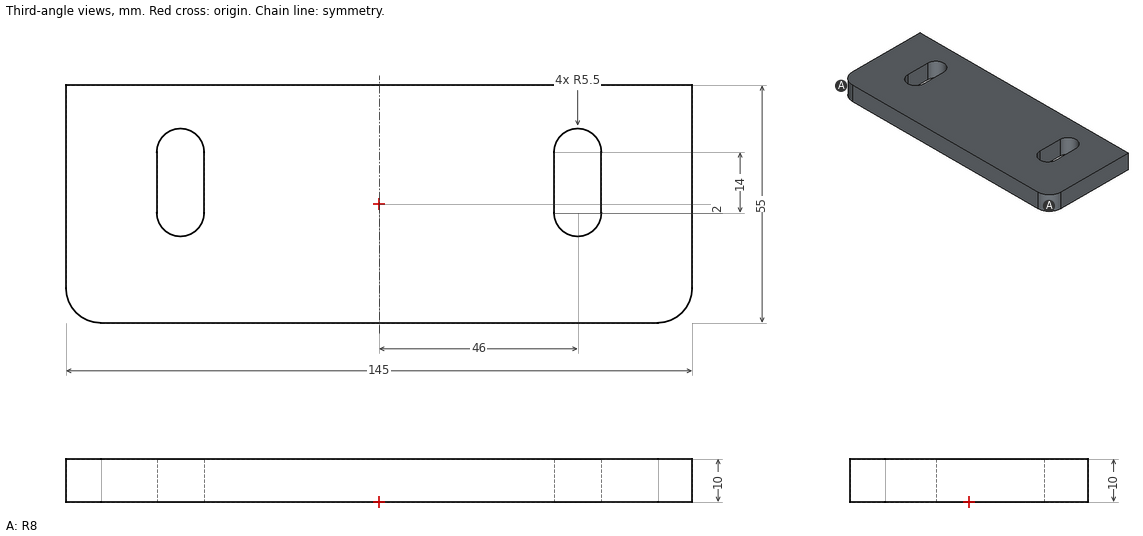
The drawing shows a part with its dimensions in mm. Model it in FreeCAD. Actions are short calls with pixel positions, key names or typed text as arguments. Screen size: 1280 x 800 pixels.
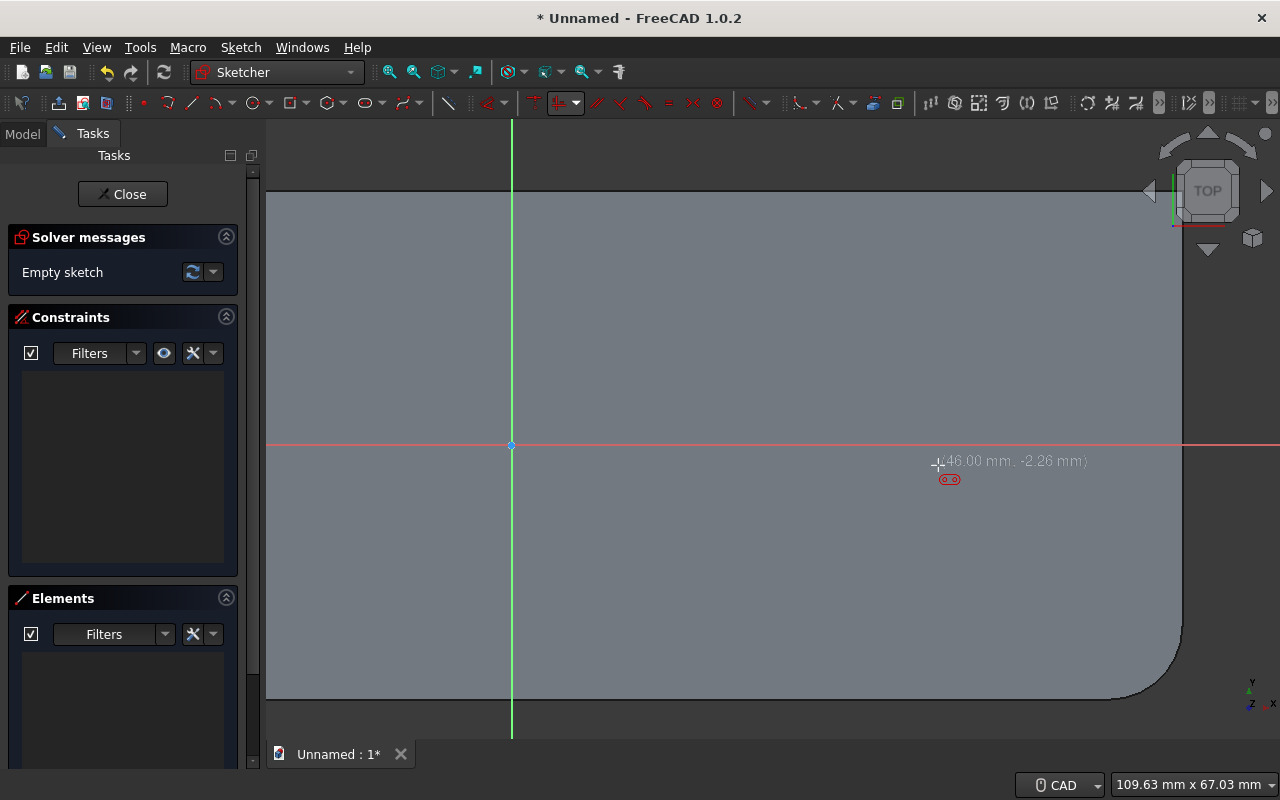
click(937, 464)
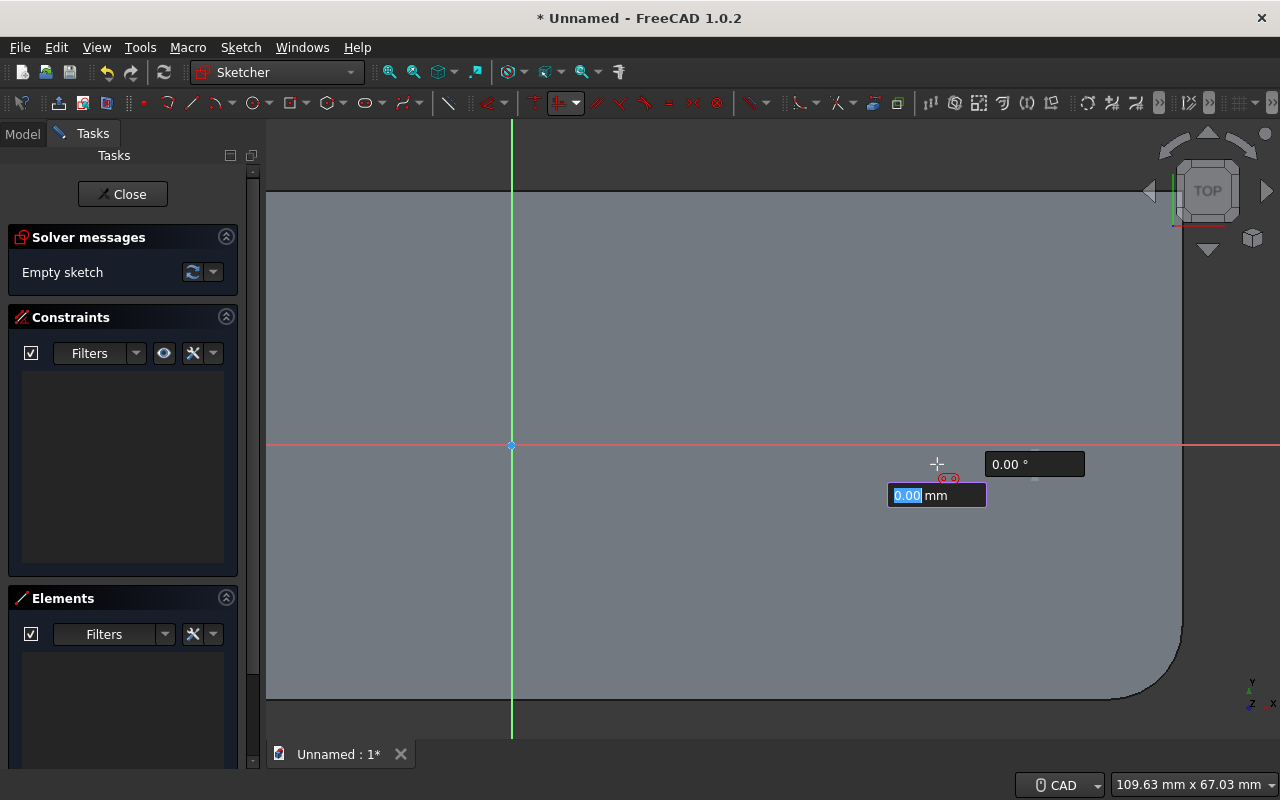
click(937, 334)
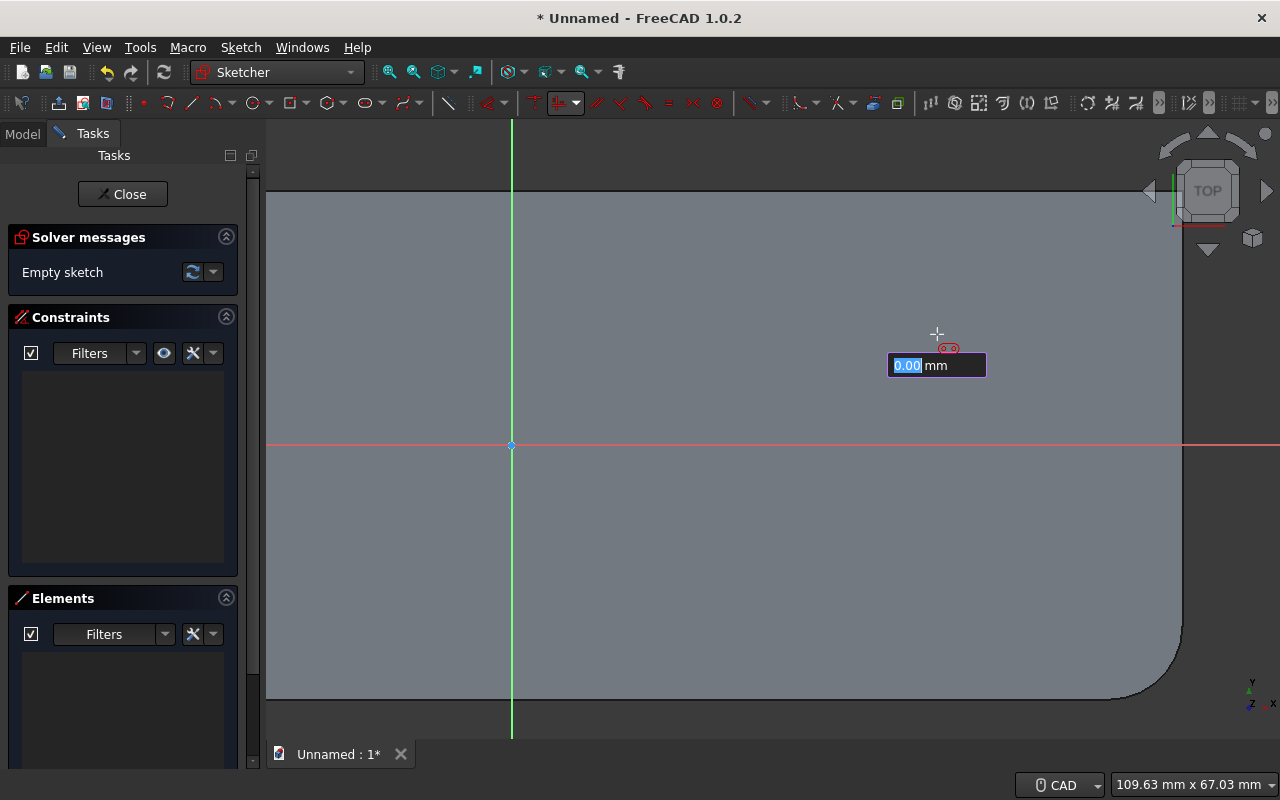
click(988, 399)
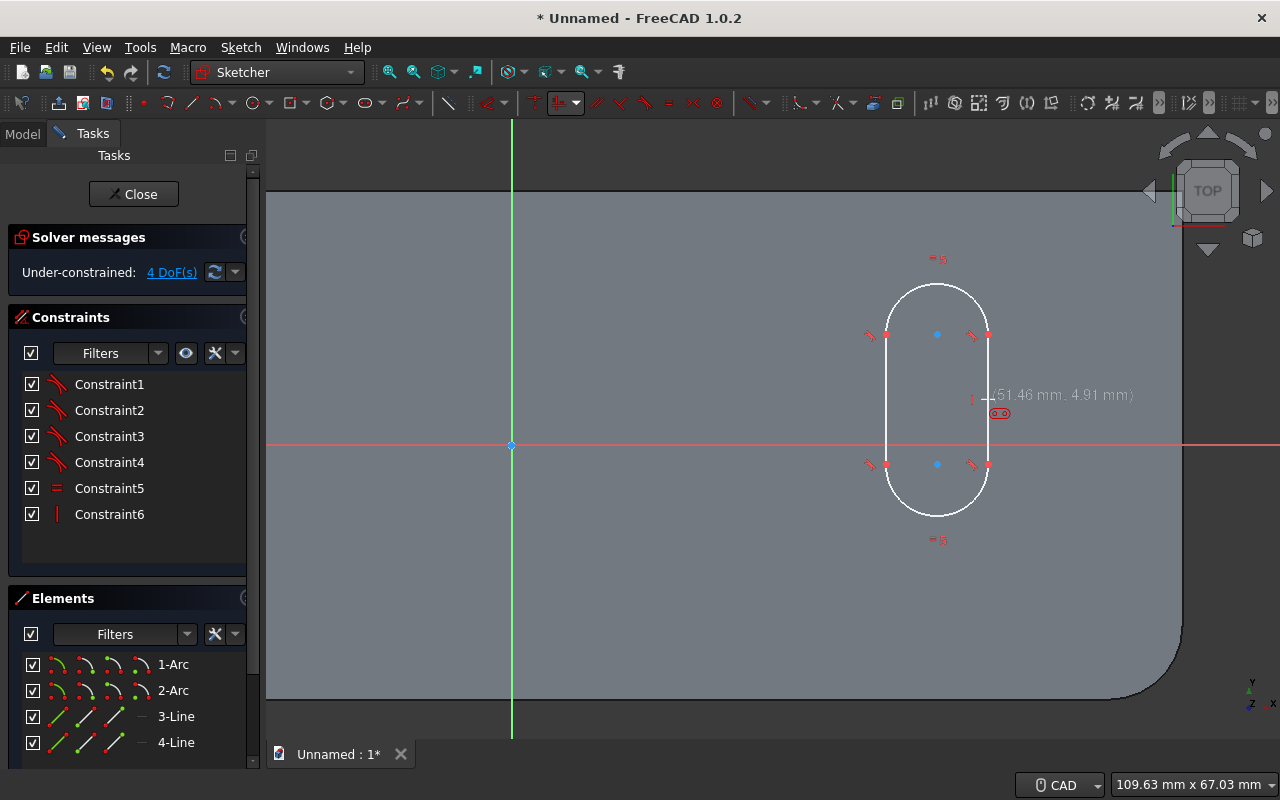
scroll(1096, 490, down, 2)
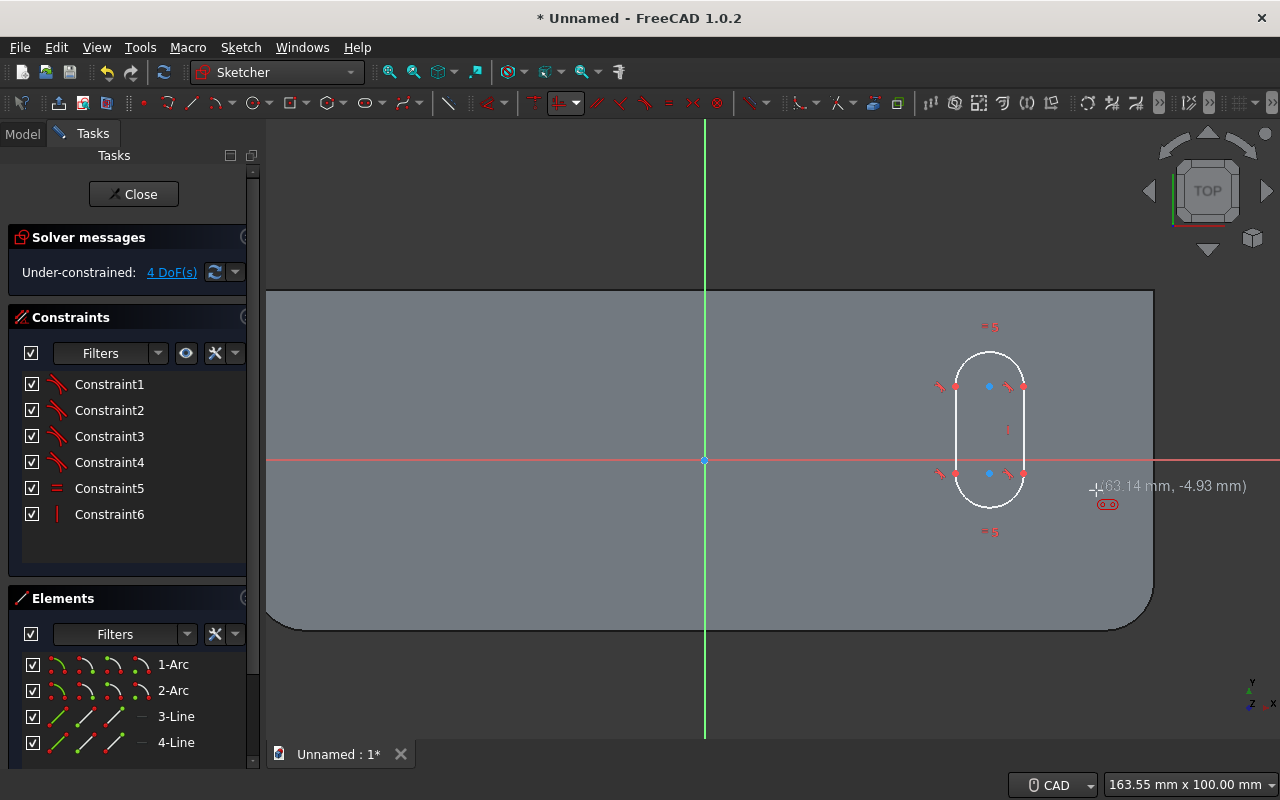
scroll(420, 473, up, 2)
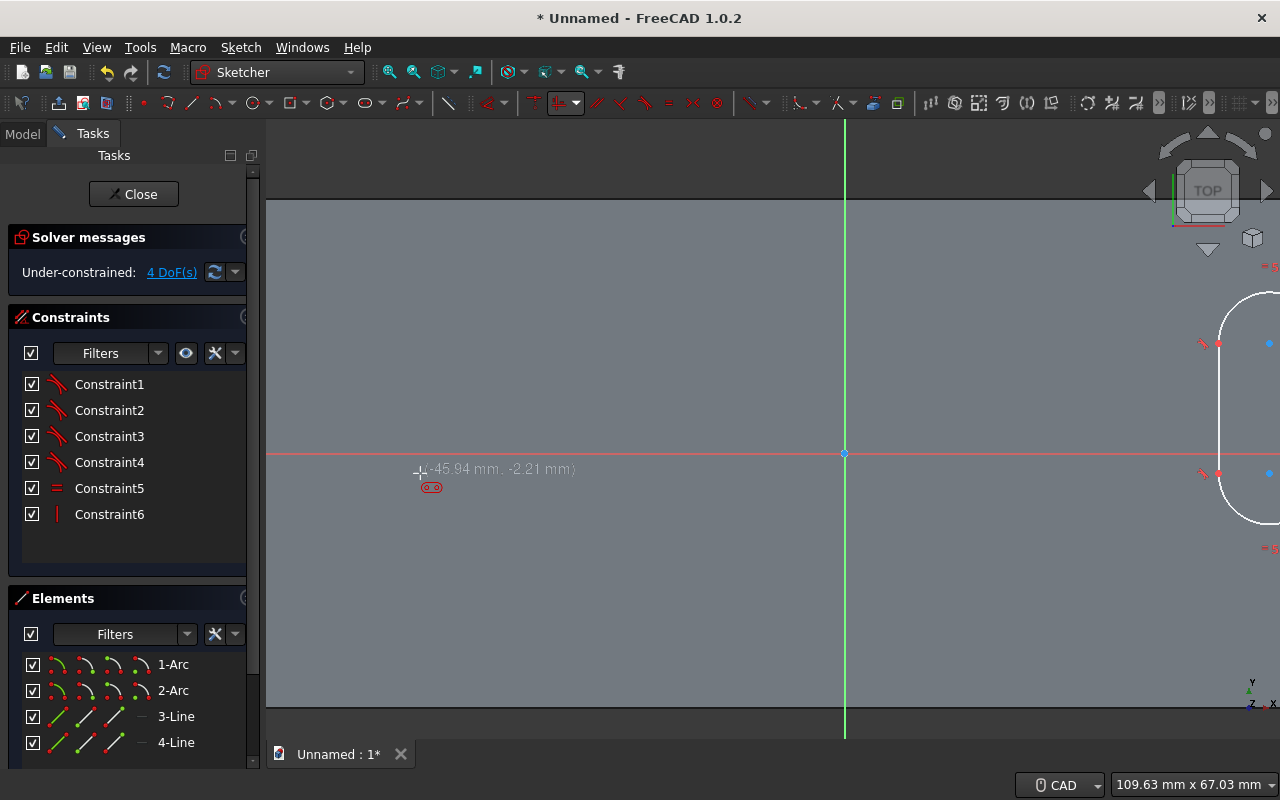
click(419, 472)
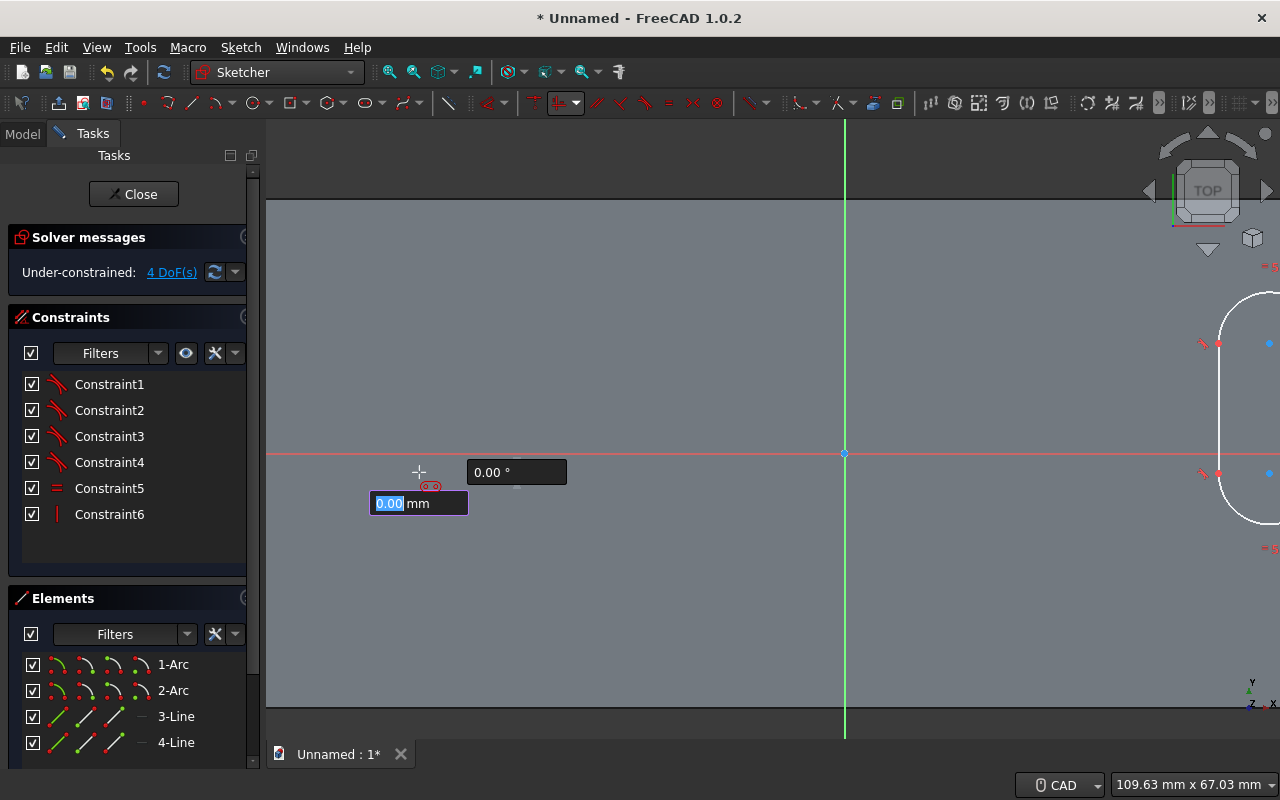
click(419, 343)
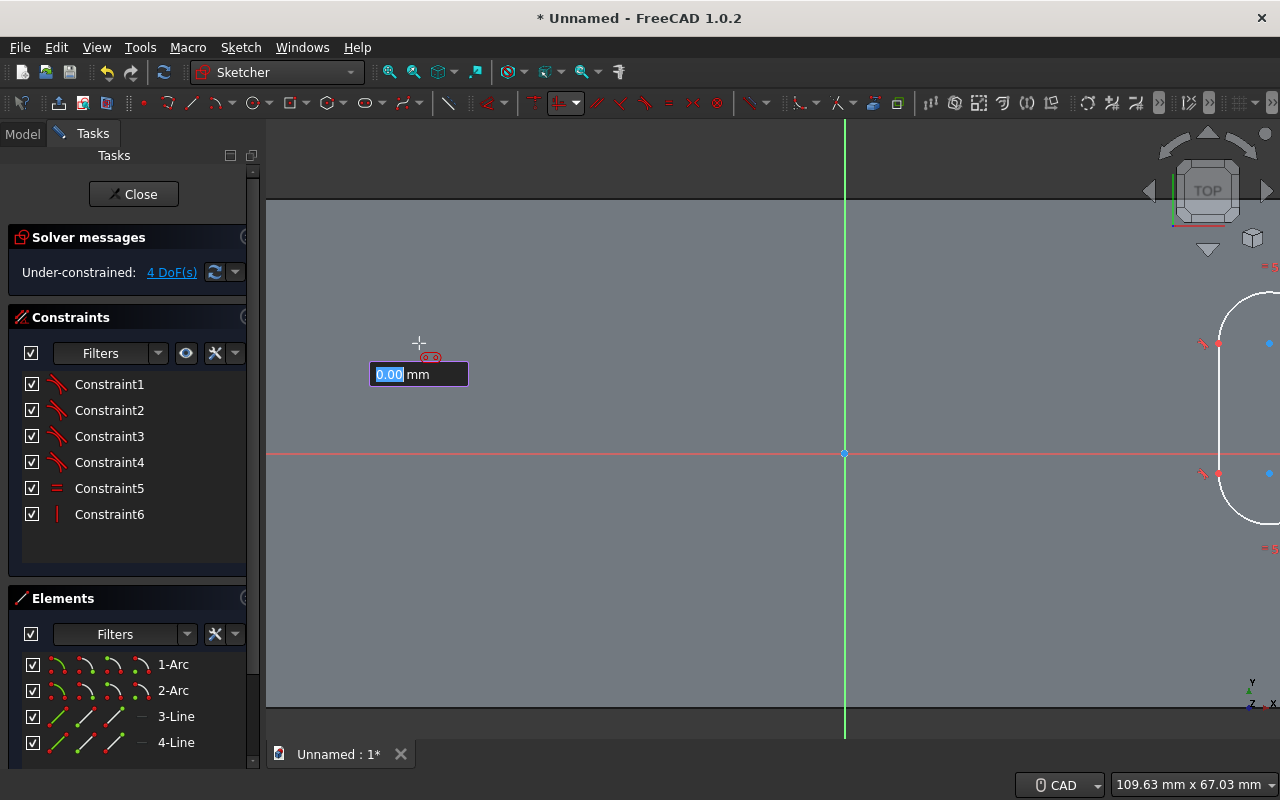
click(470, 408)
key(Escape)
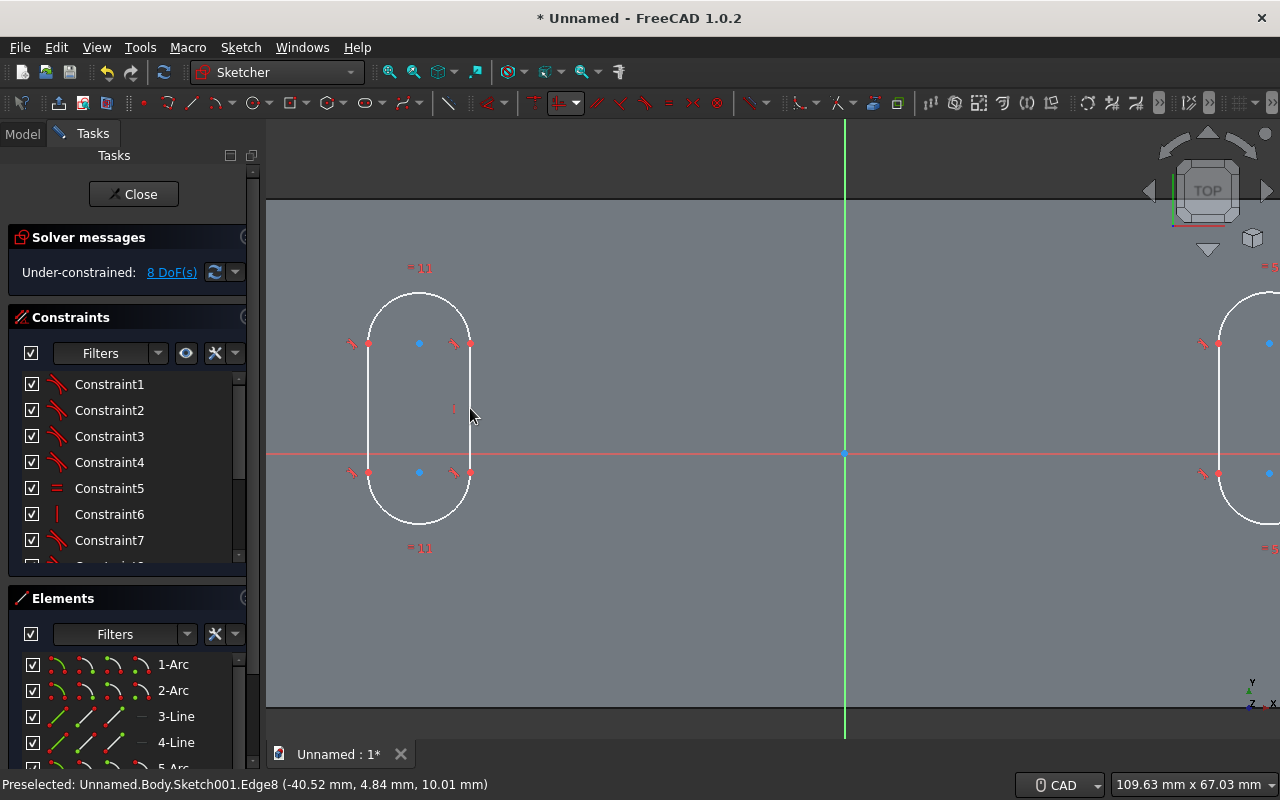
scroll(419, 473, down, 2)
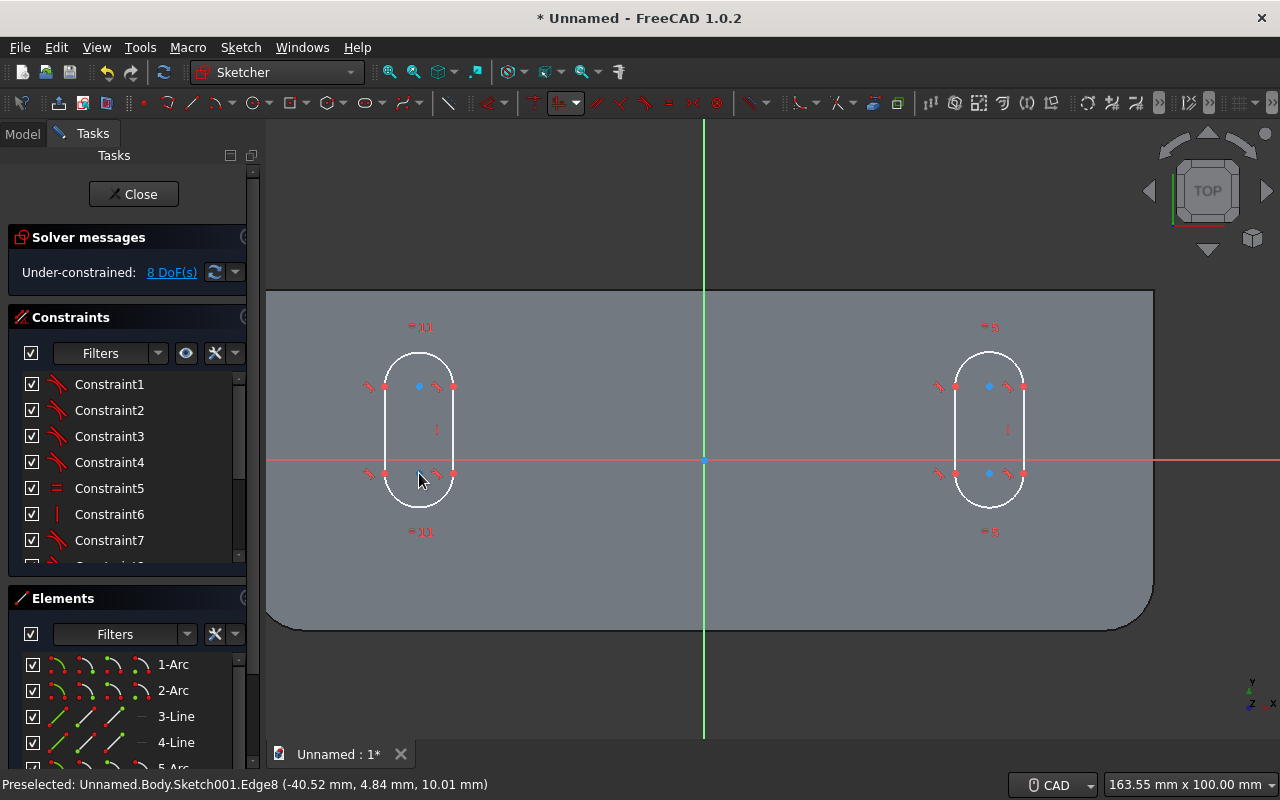
click(969, 501)